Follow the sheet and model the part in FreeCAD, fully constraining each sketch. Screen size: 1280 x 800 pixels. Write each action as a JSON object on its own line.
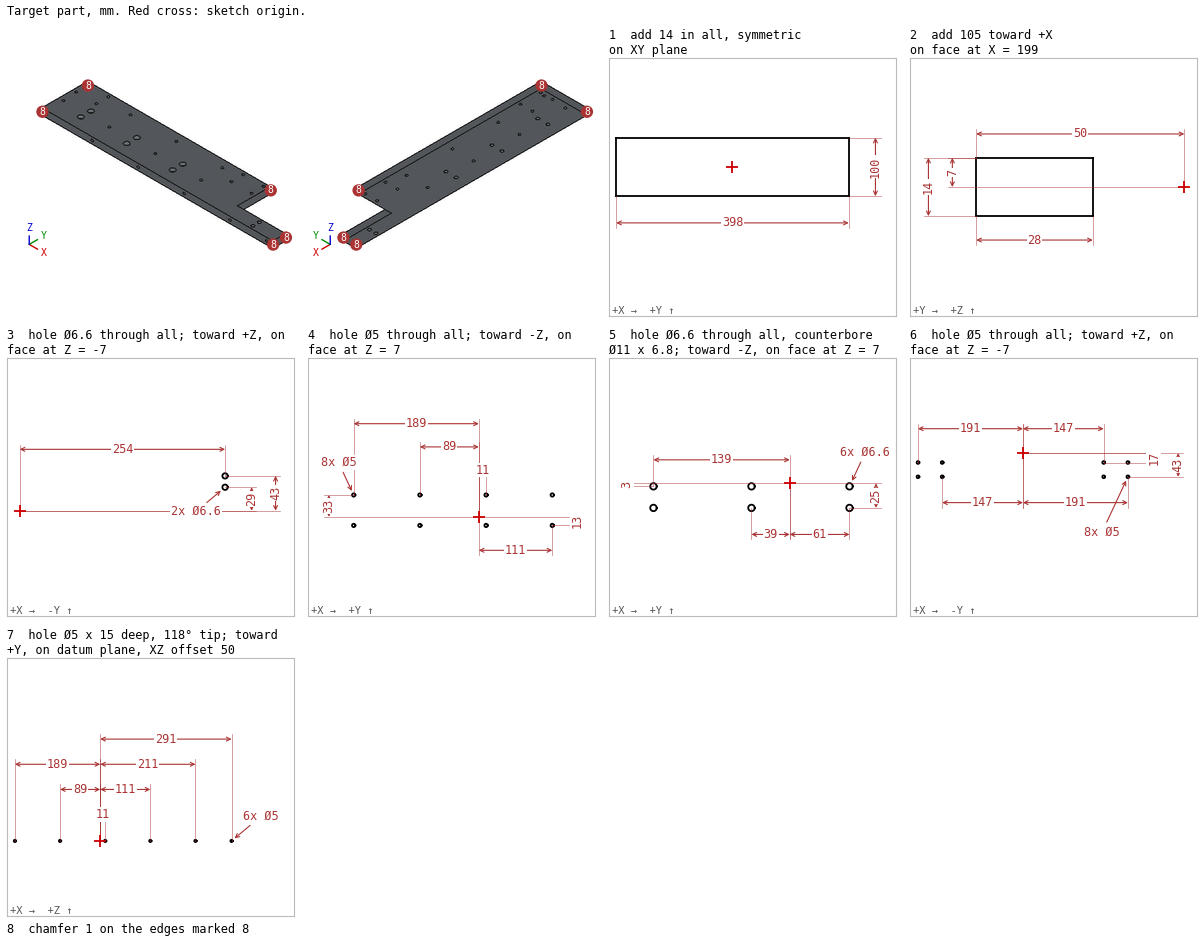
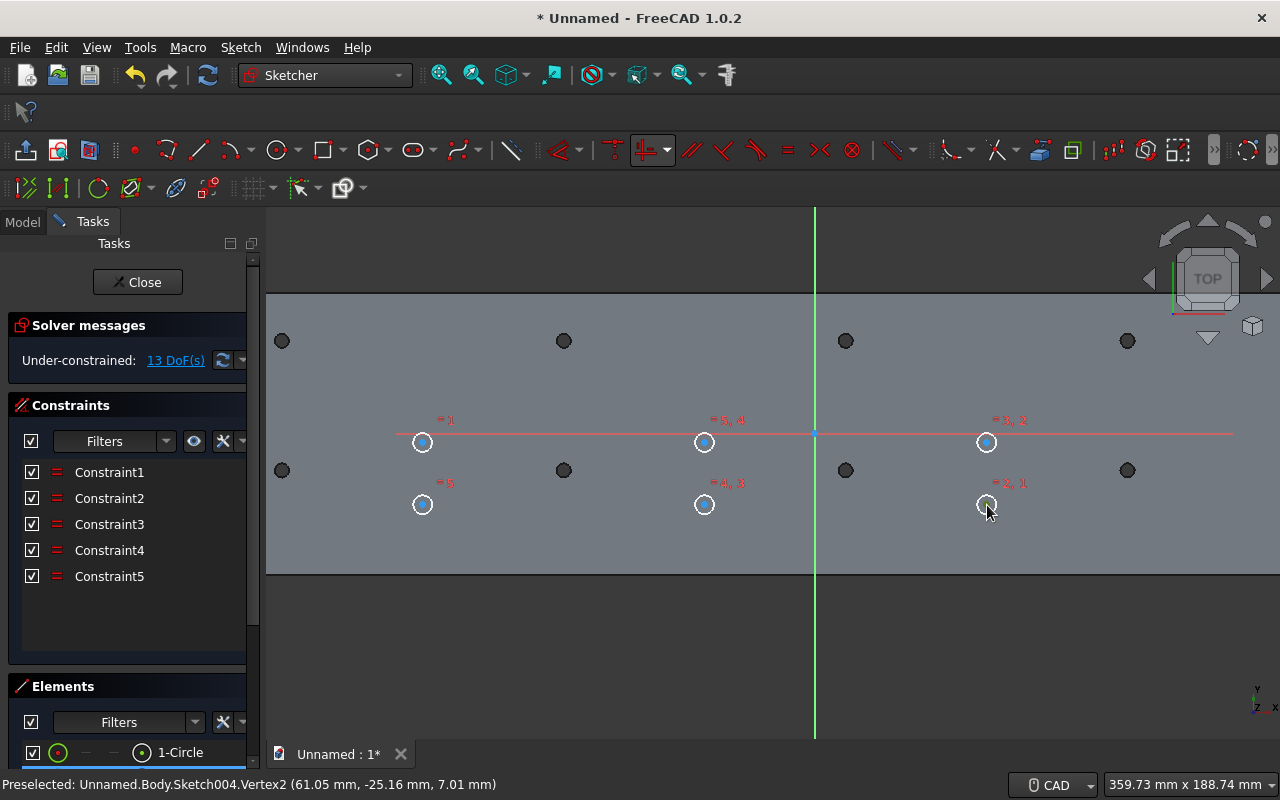
{"action": "left_click", "coordinate": [987, 443]}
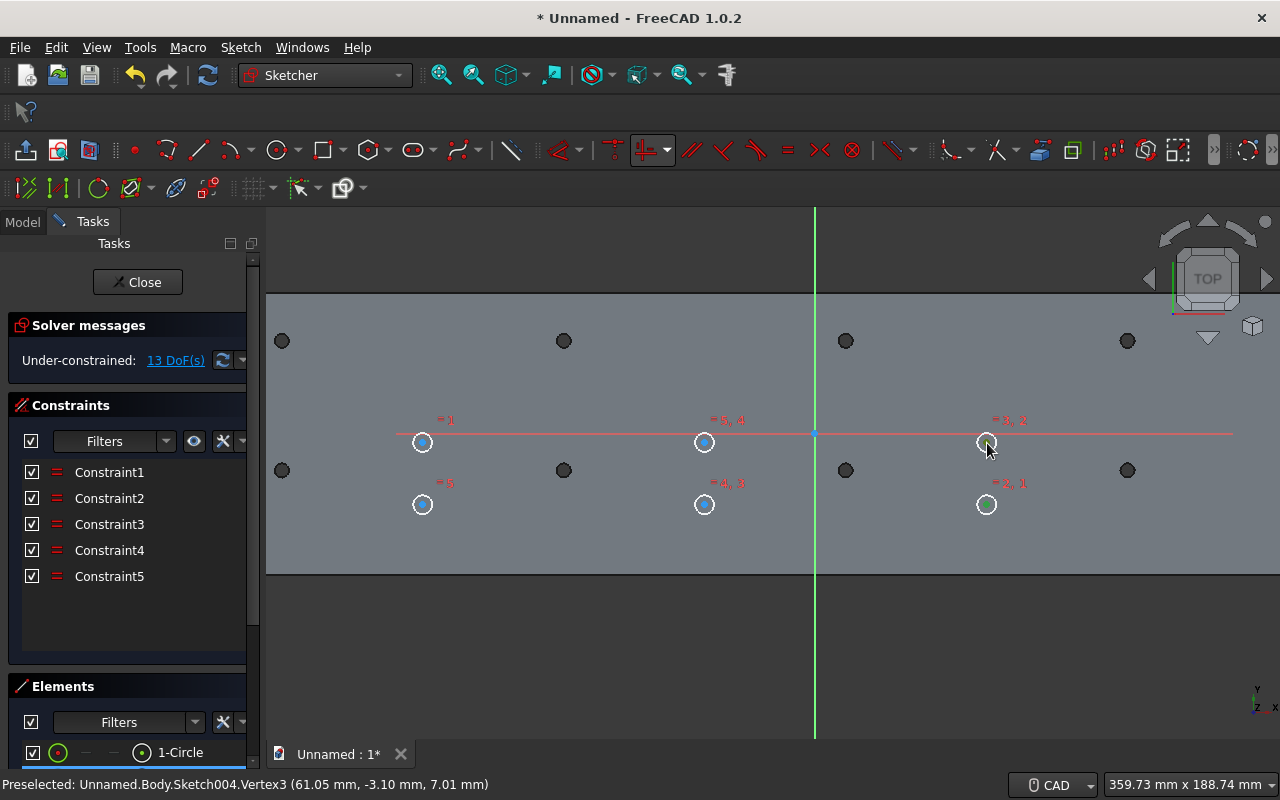
{"action": "key", "text": "v"}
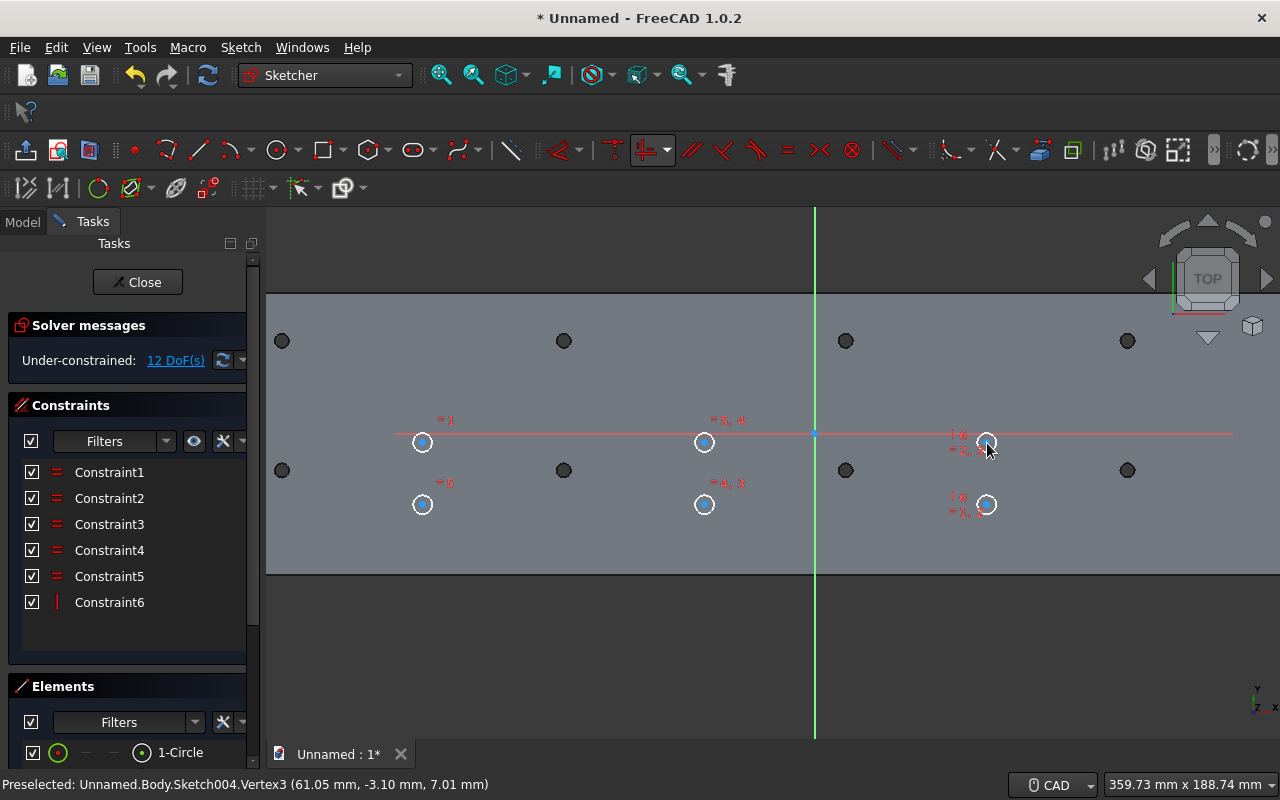
{"action": "left_click", "coordinate": [423, 443]}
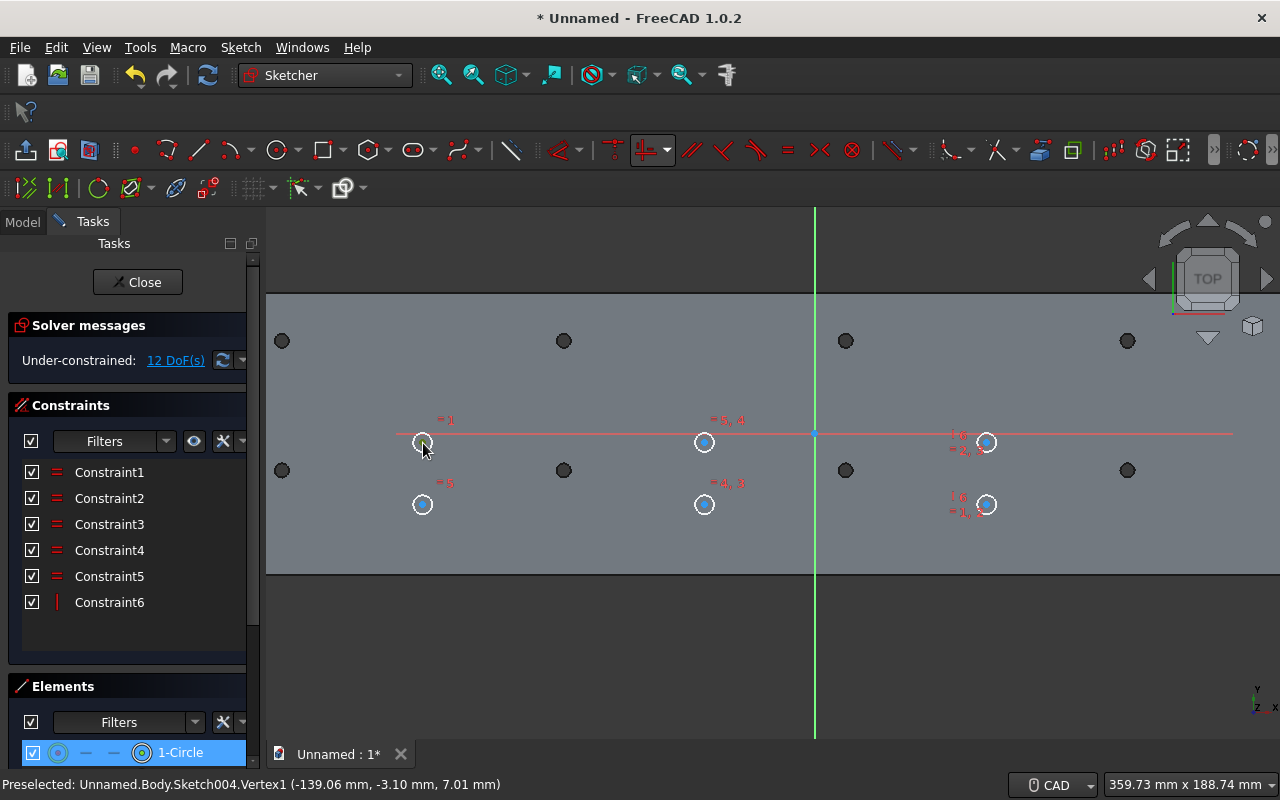
{"action": "left_click", "coordinate": [987, 443]}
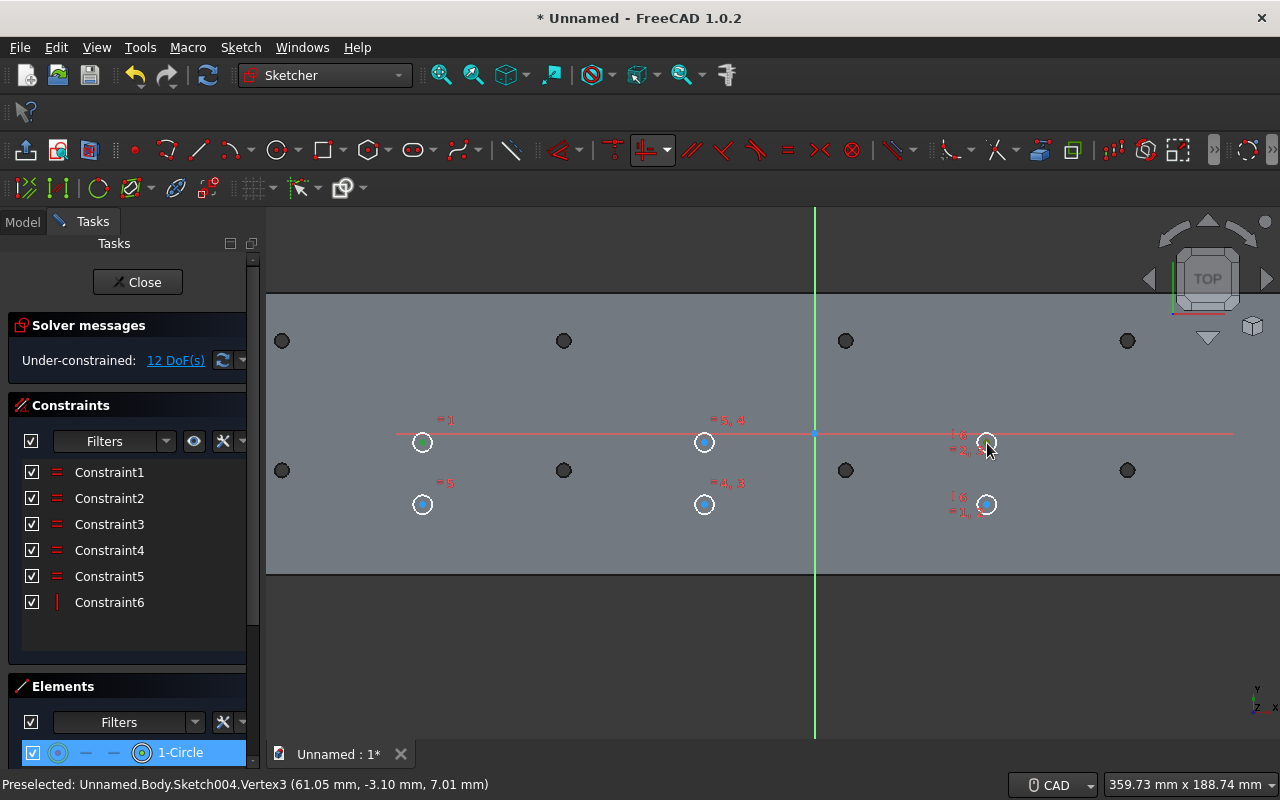
{"action": "key", "text": "h"}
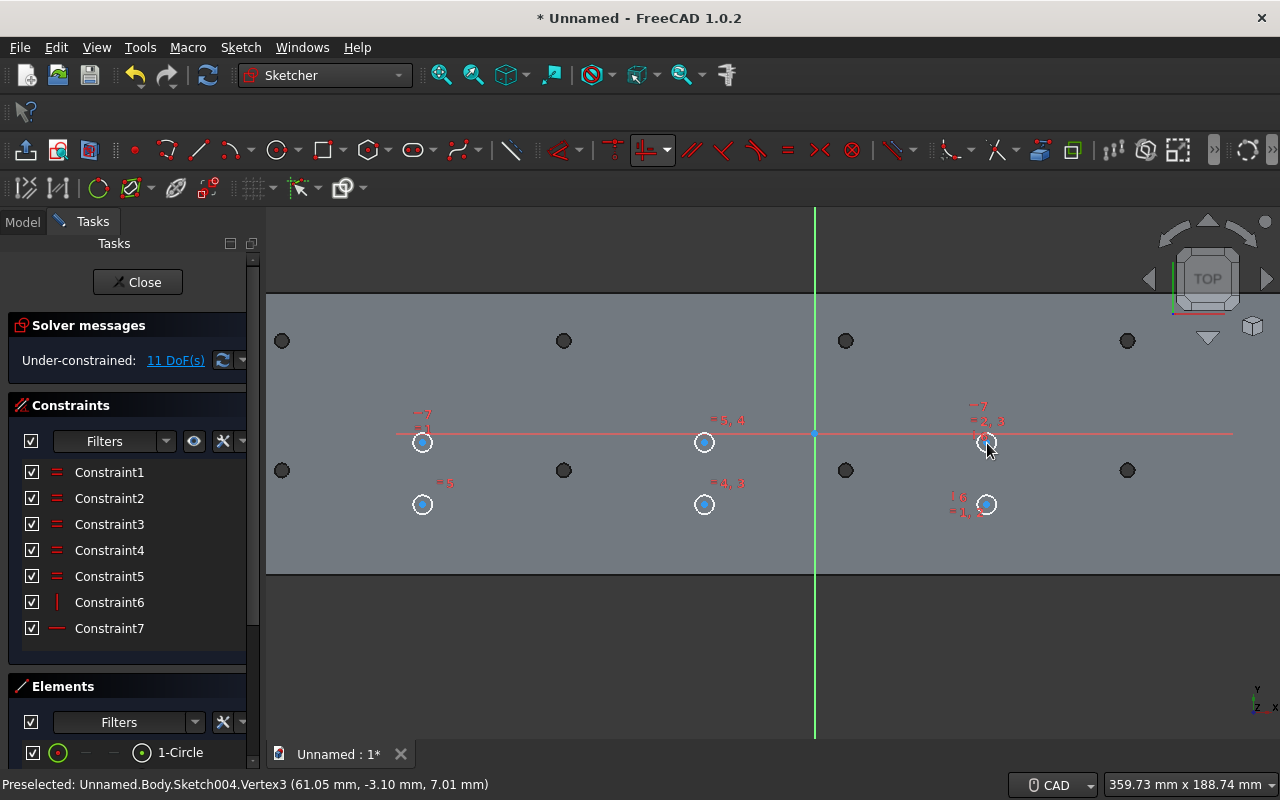
{"action": "left_click", "coordinate": [987, 505]}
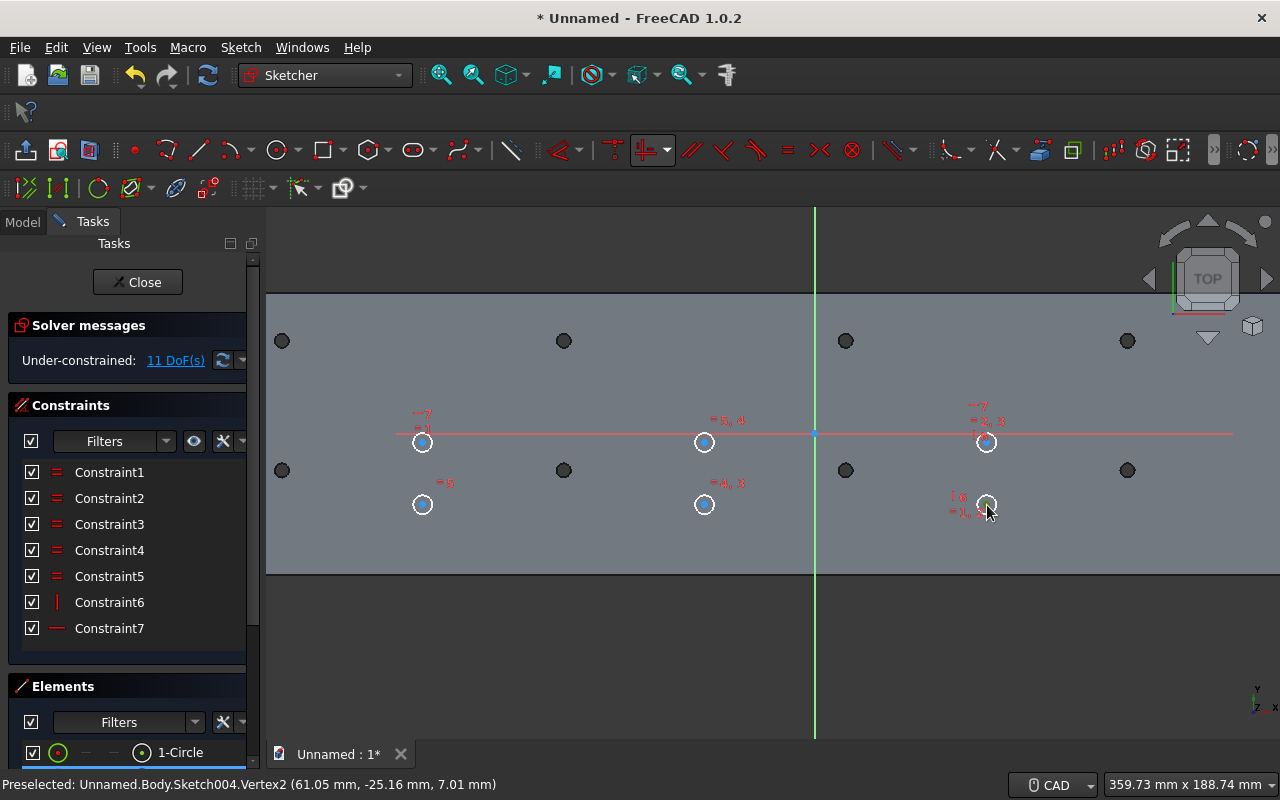
{"action": "left_click", "coordinate": [705, 505]}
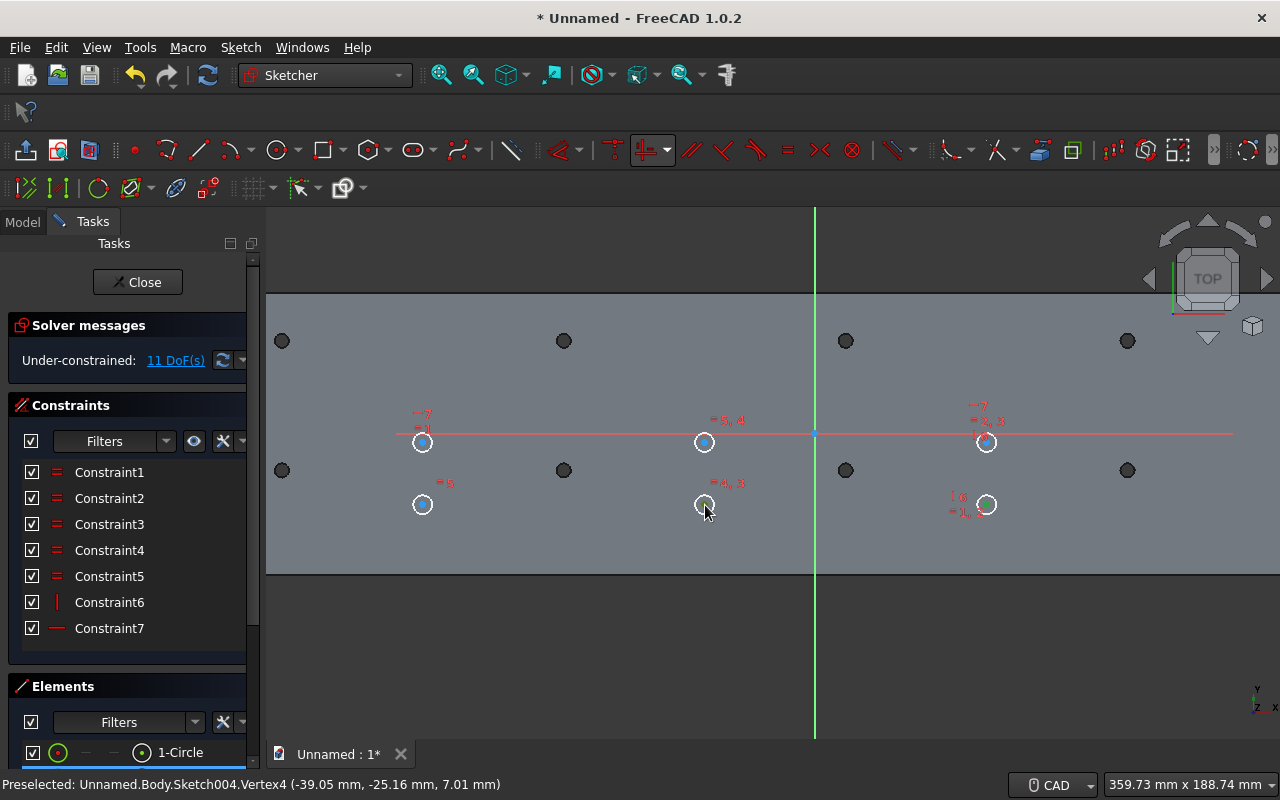
{"action": "left_click", "coordinate": [670, 150]}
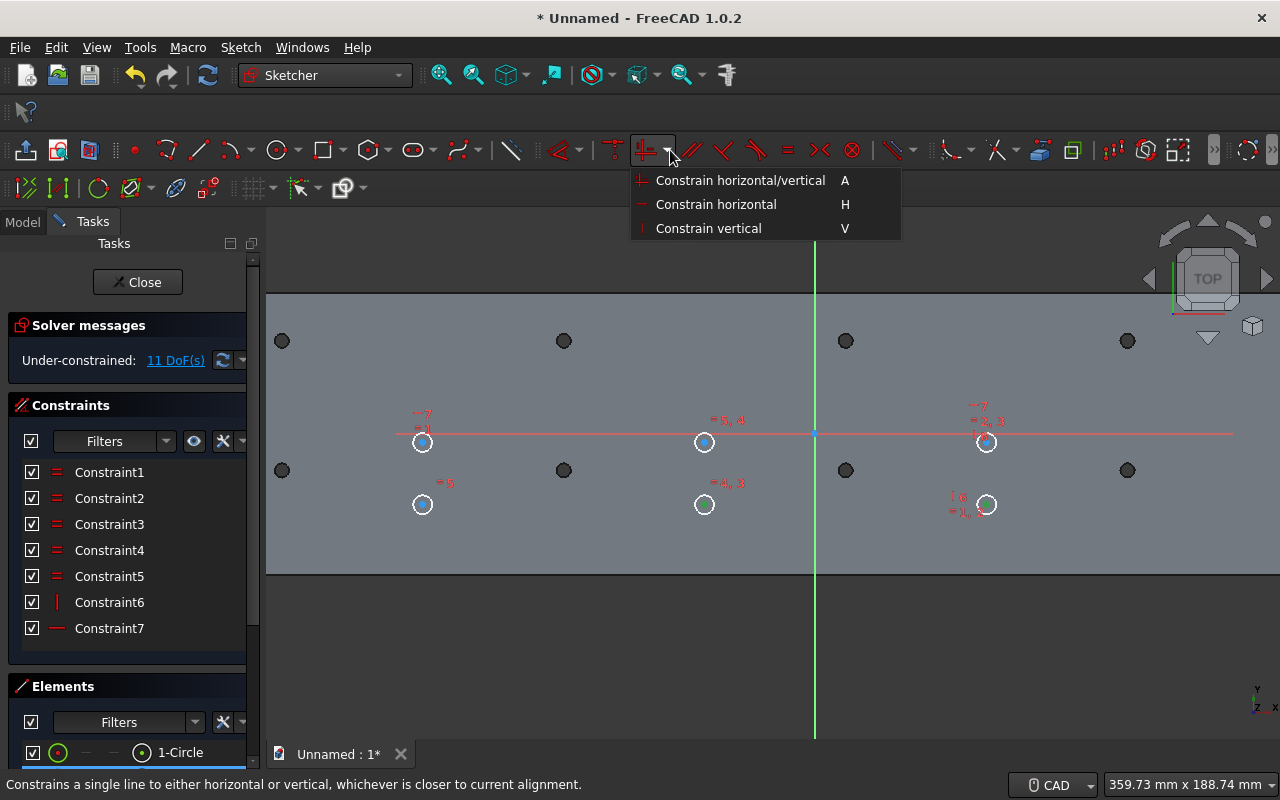
{"action": "left_click", "coordinate": [766, 204]}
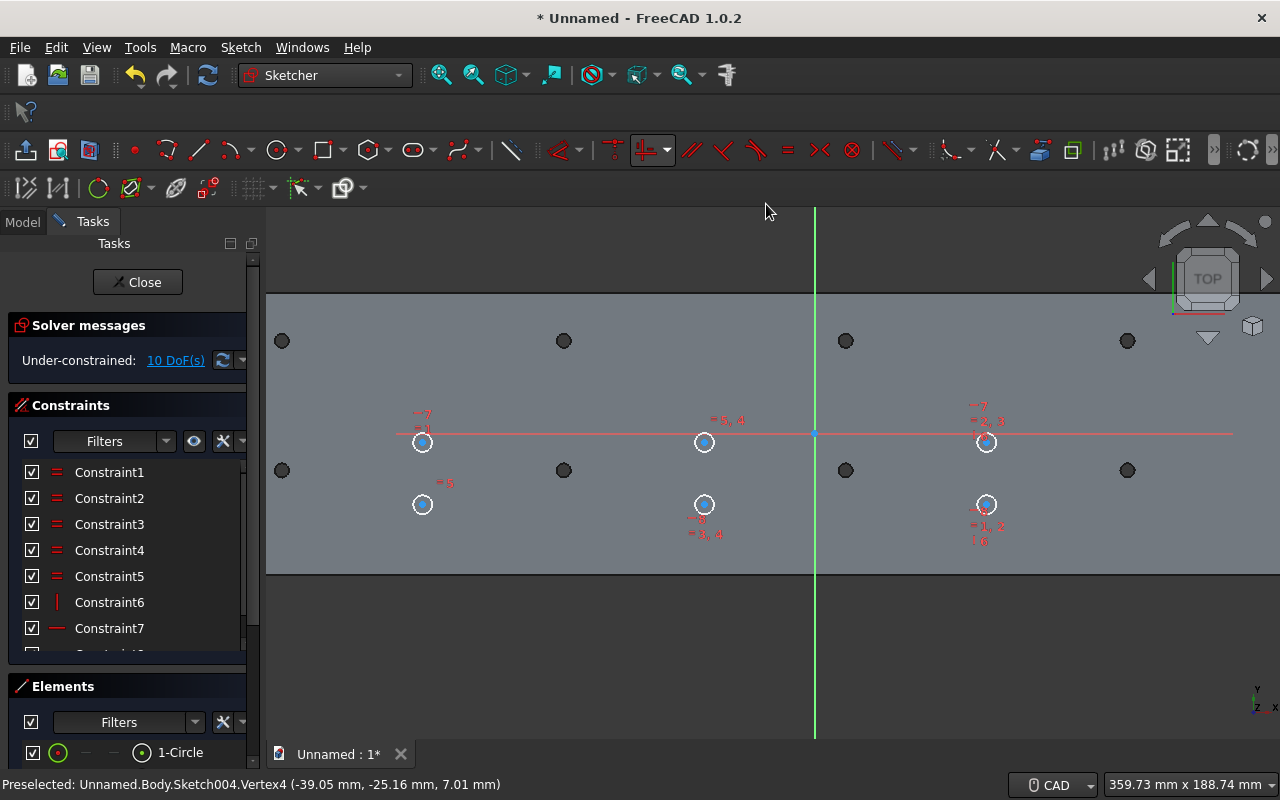
{"action": "left_click", "coordinate": [705, 505]}